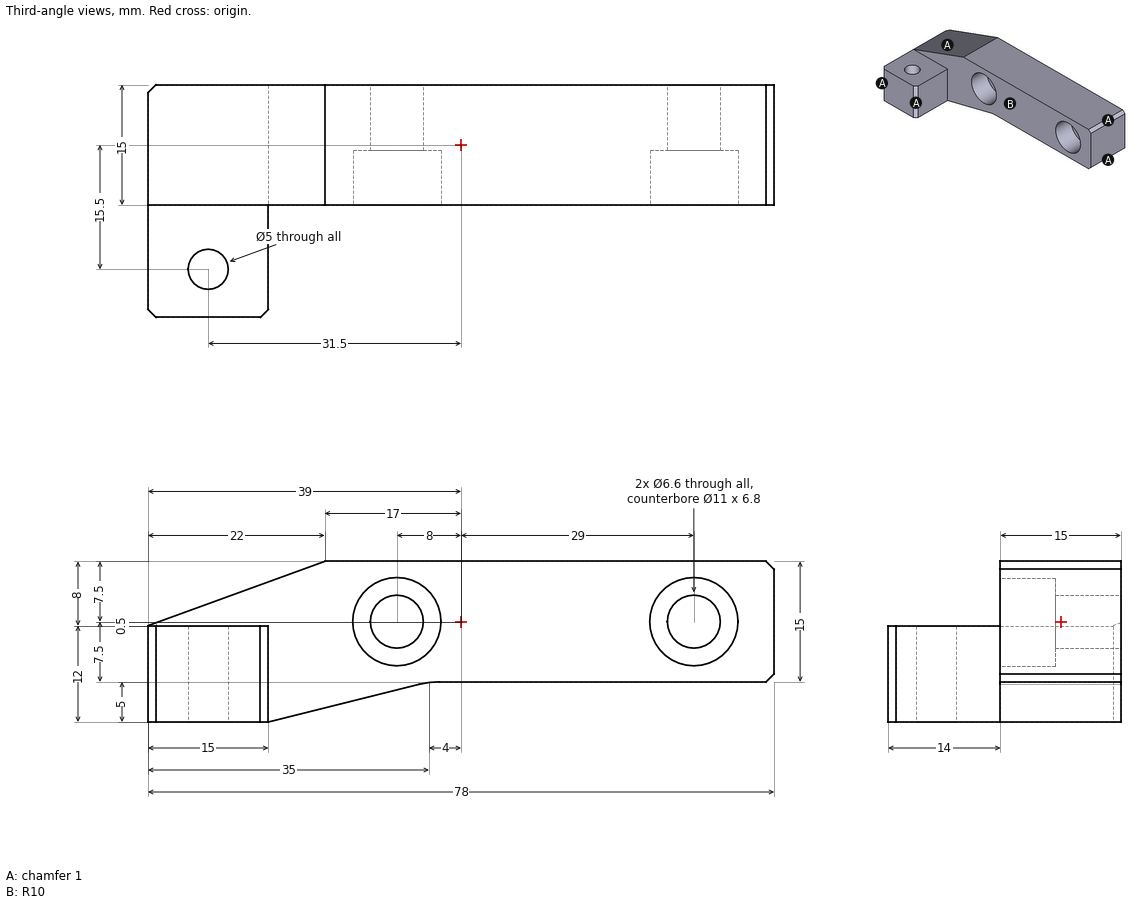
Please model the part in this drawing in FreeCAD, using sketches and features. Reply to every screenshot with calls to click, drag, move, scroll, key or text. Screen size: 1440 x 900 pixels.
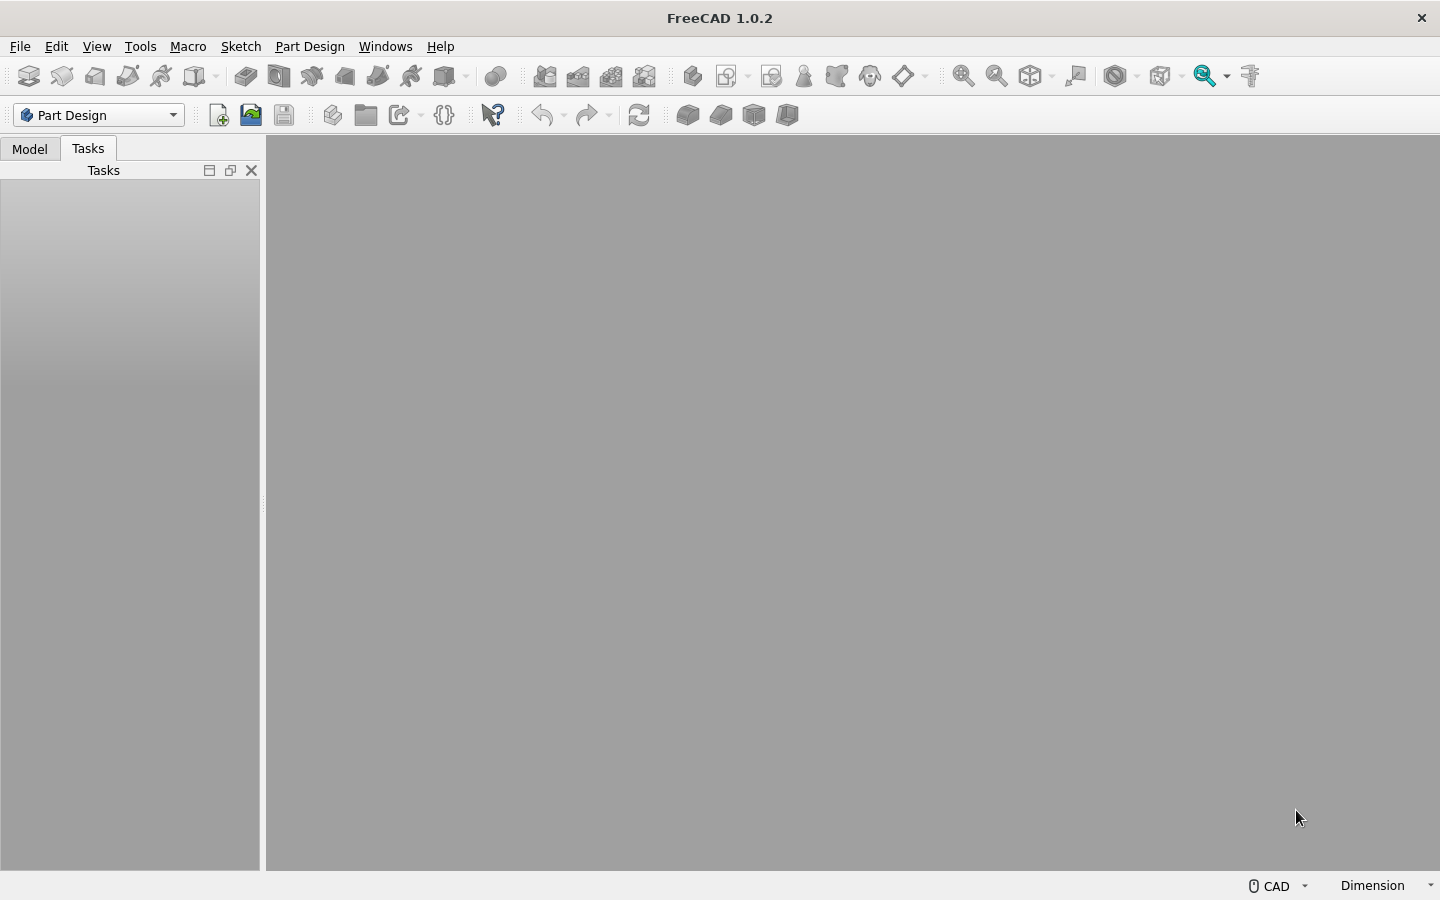
click(218, 116)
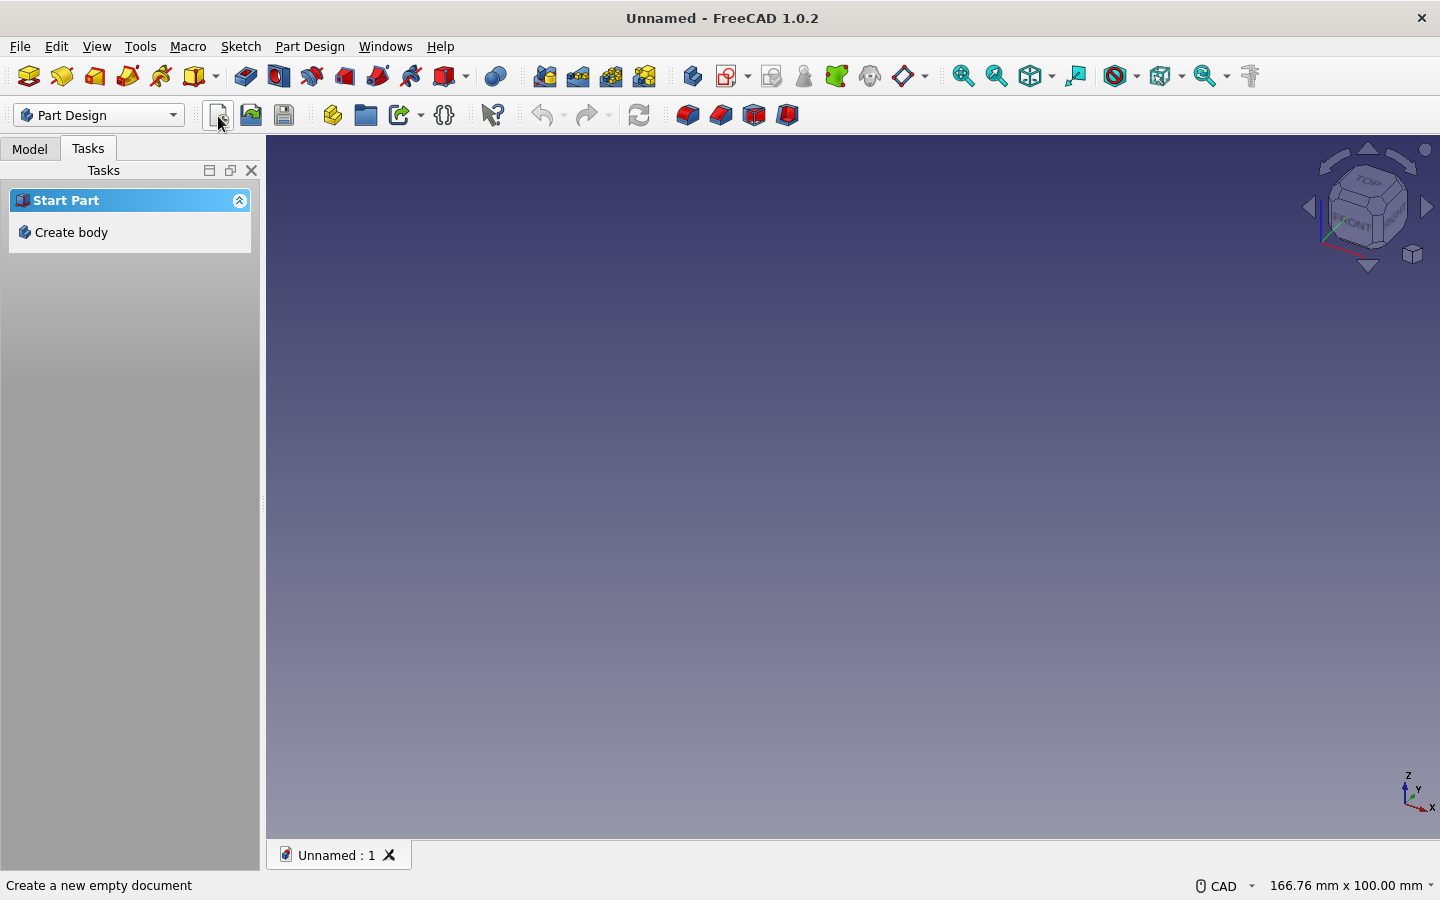
click(726, 76)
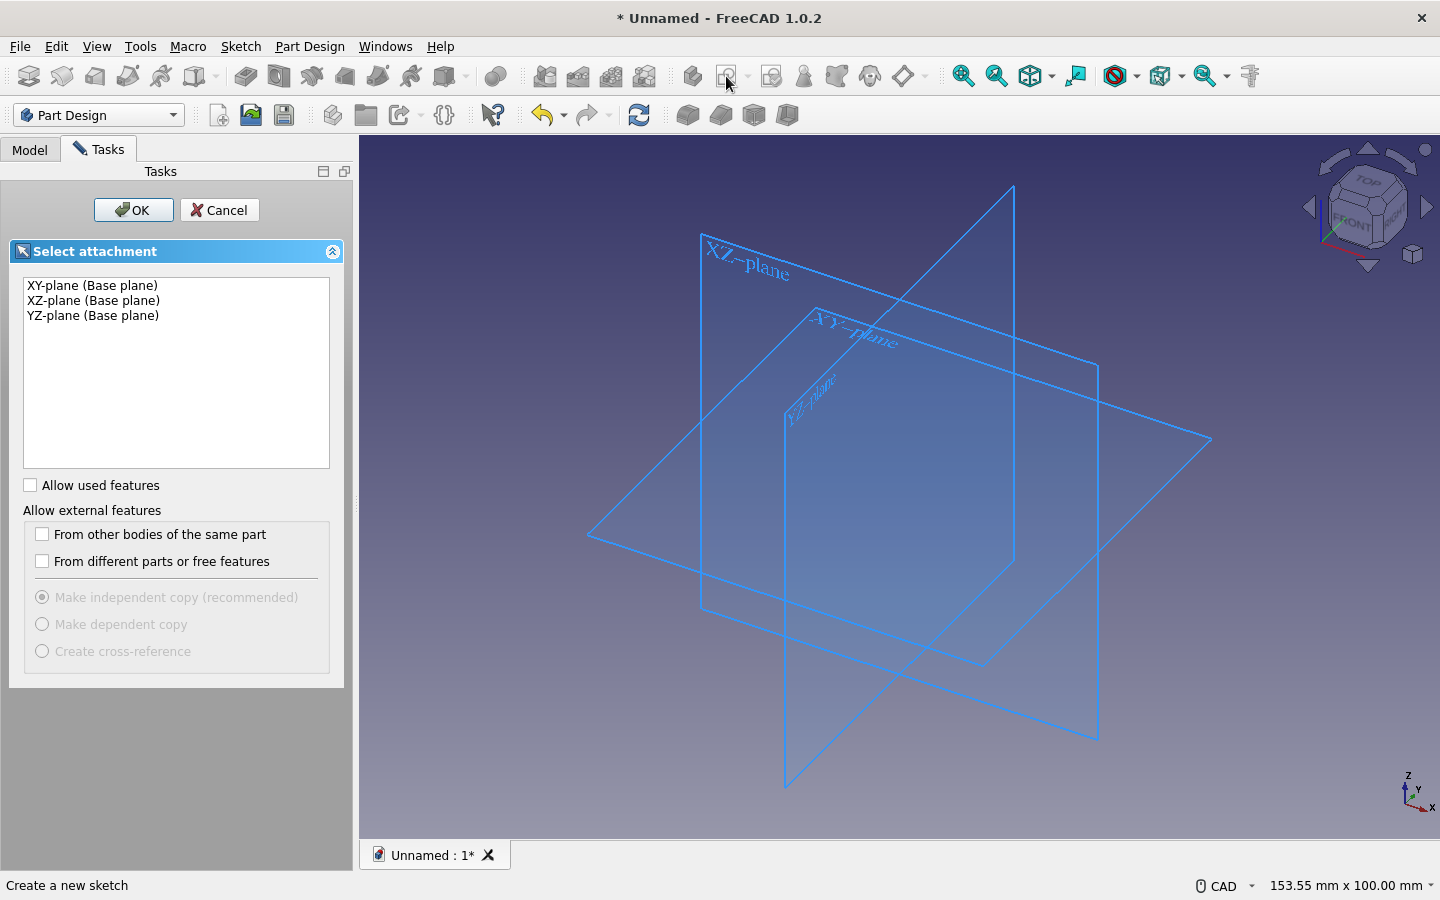
click(84, 300)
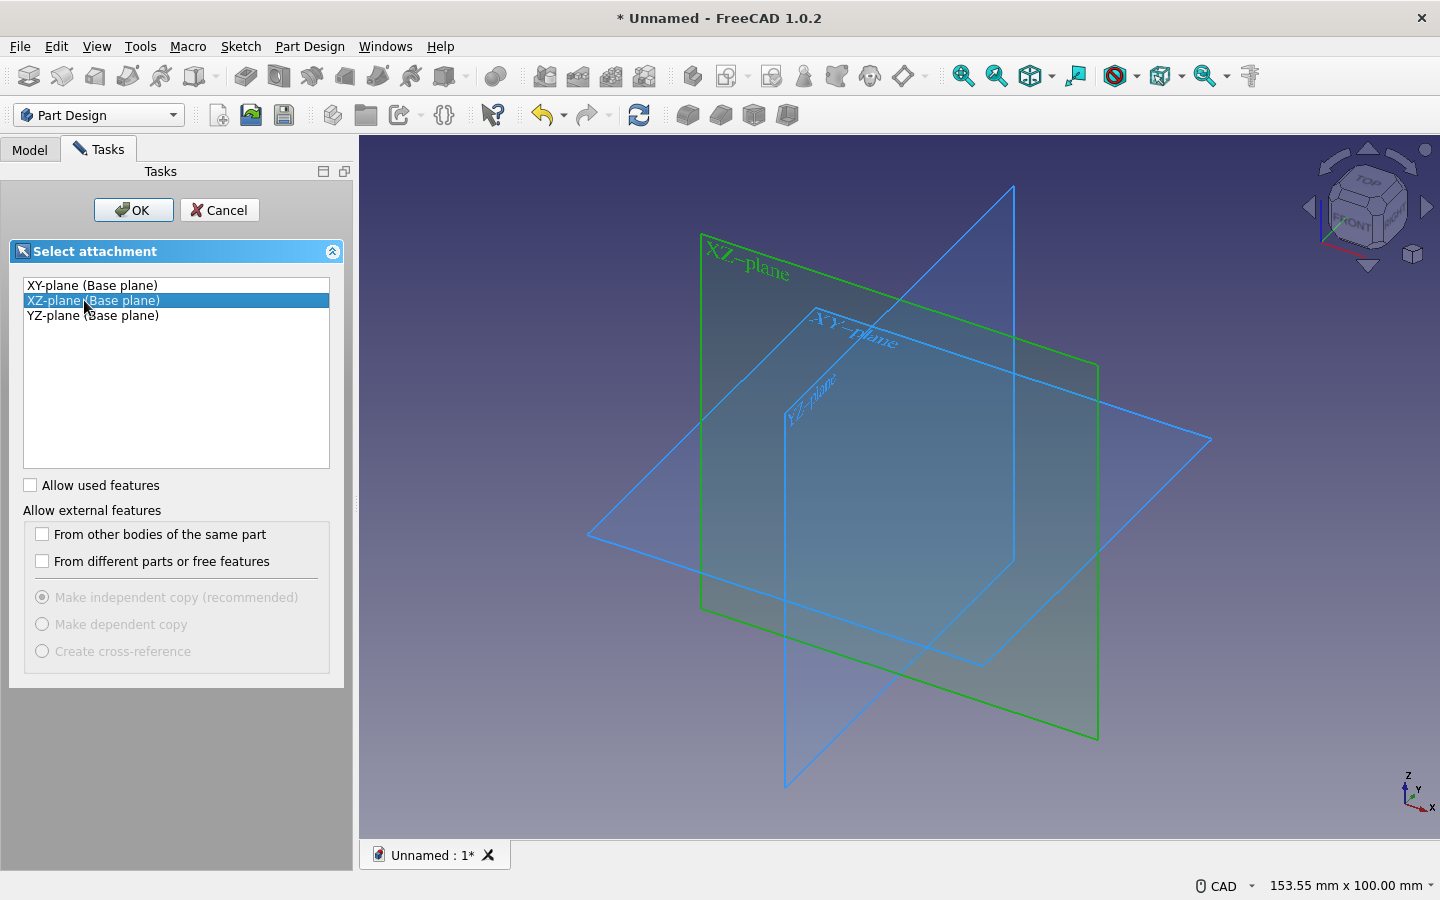
click(134, 210)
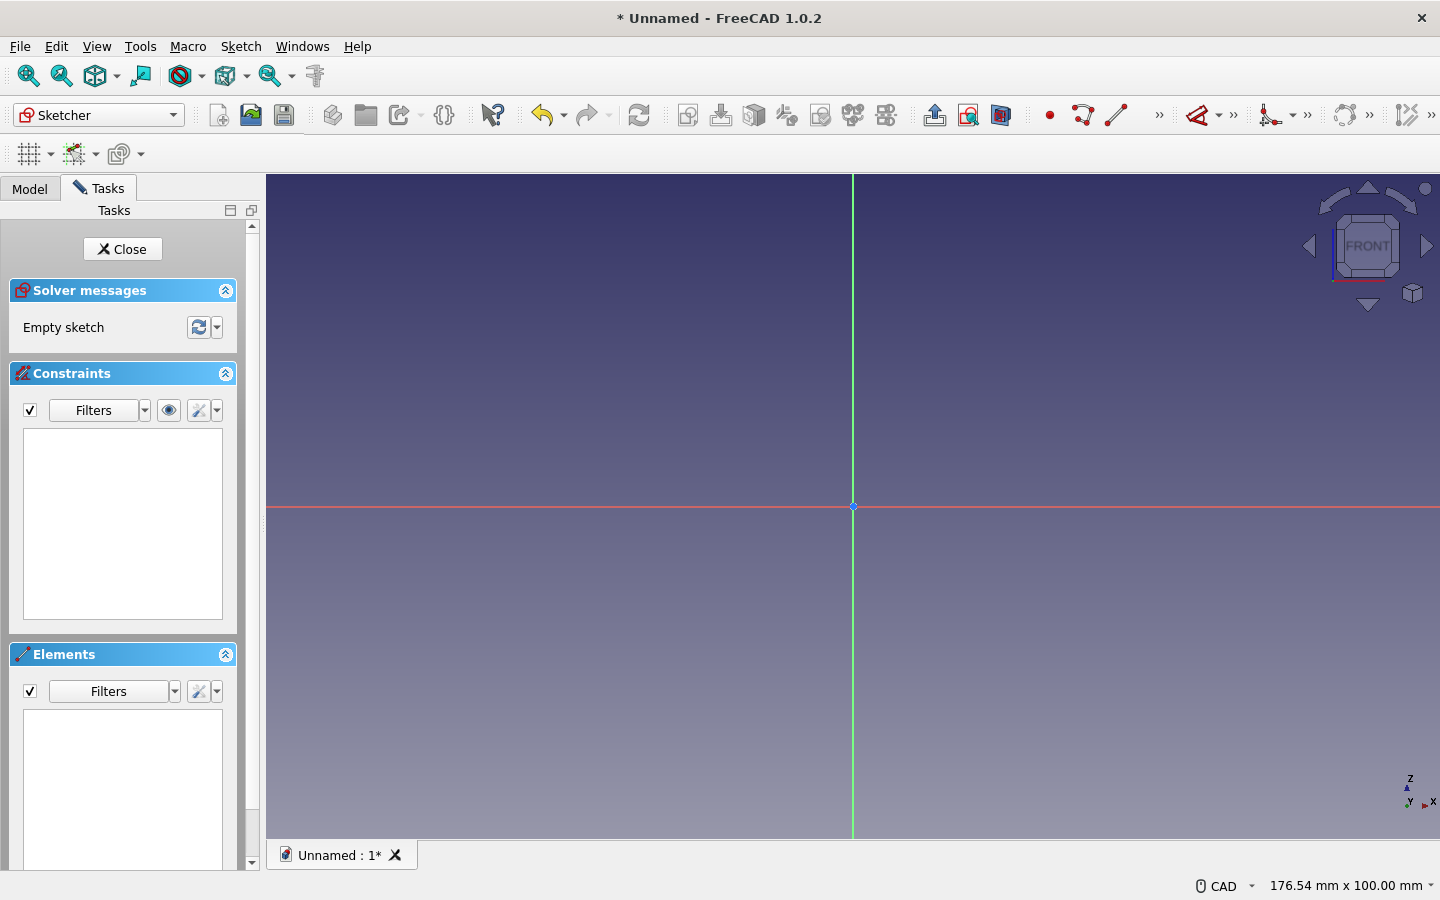
key(g)
key(v)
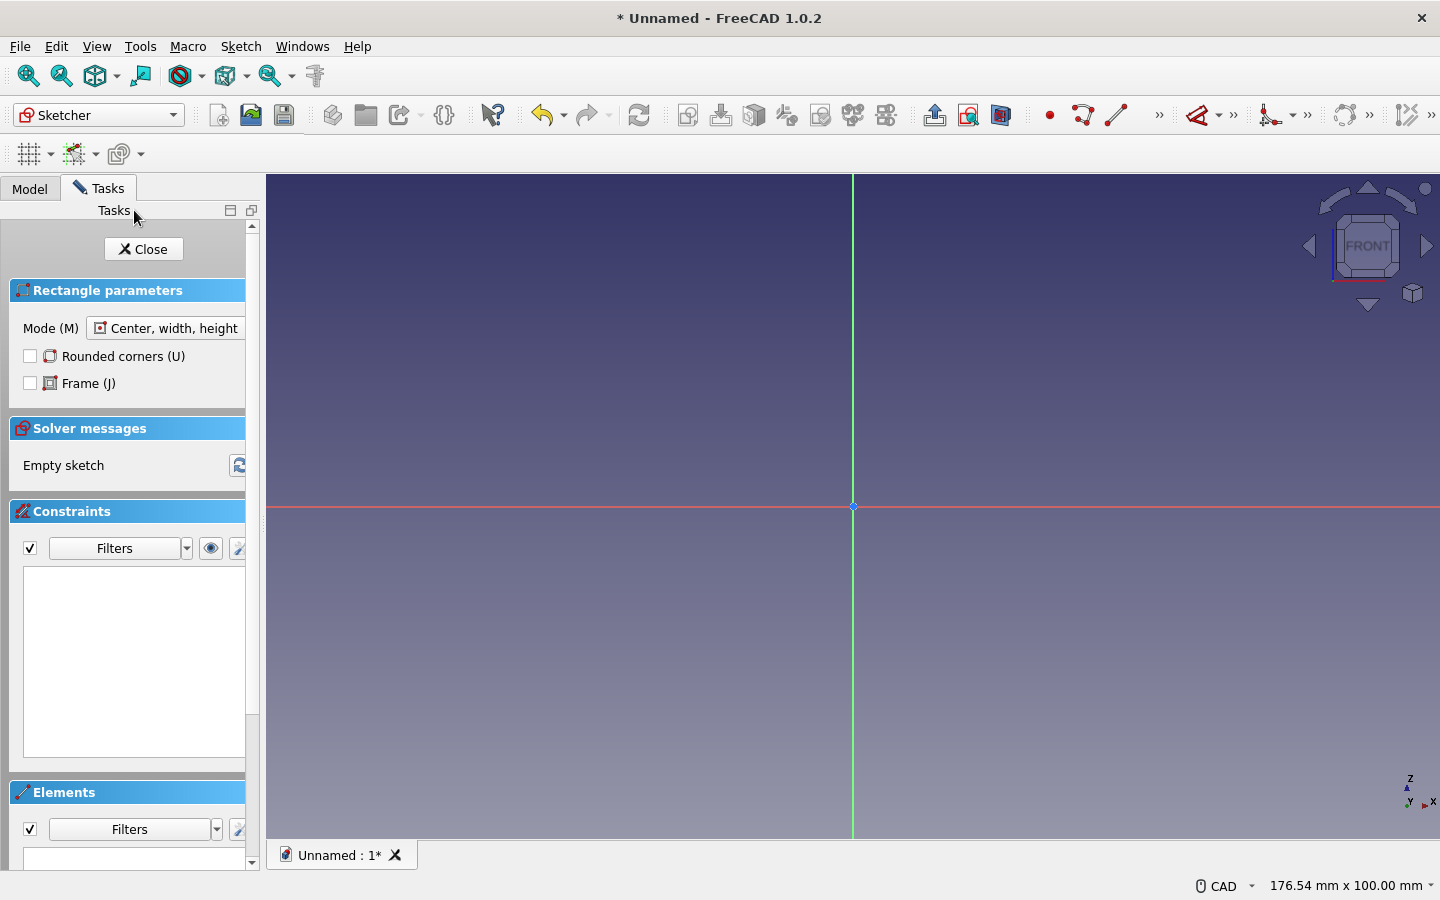
click(853, 506)
move(1112, 457)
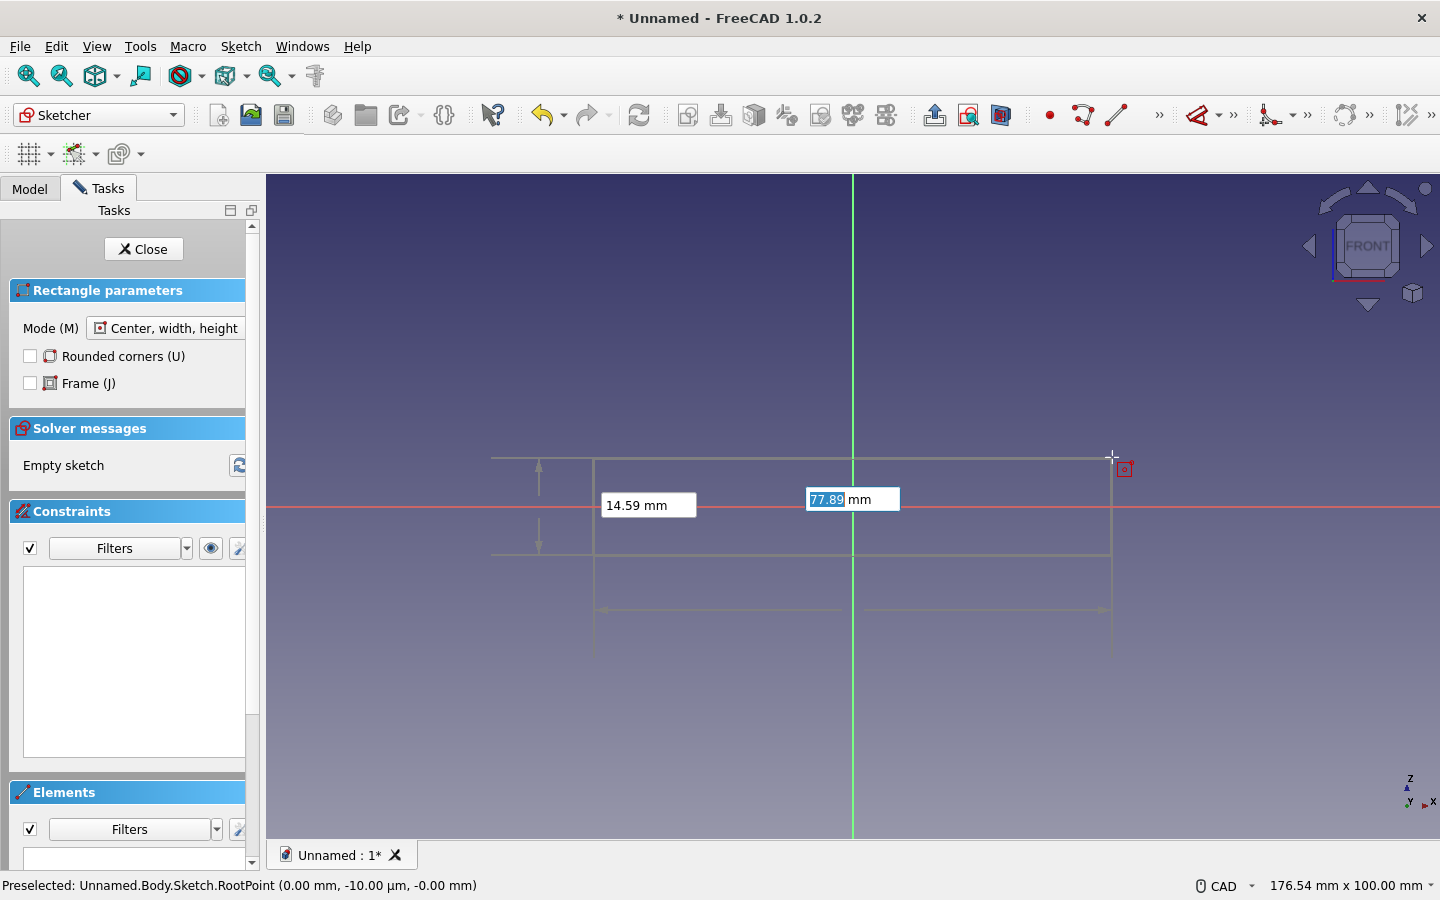
text(78)
key(Tab)
text(15)
key(Return)
key(Escape)